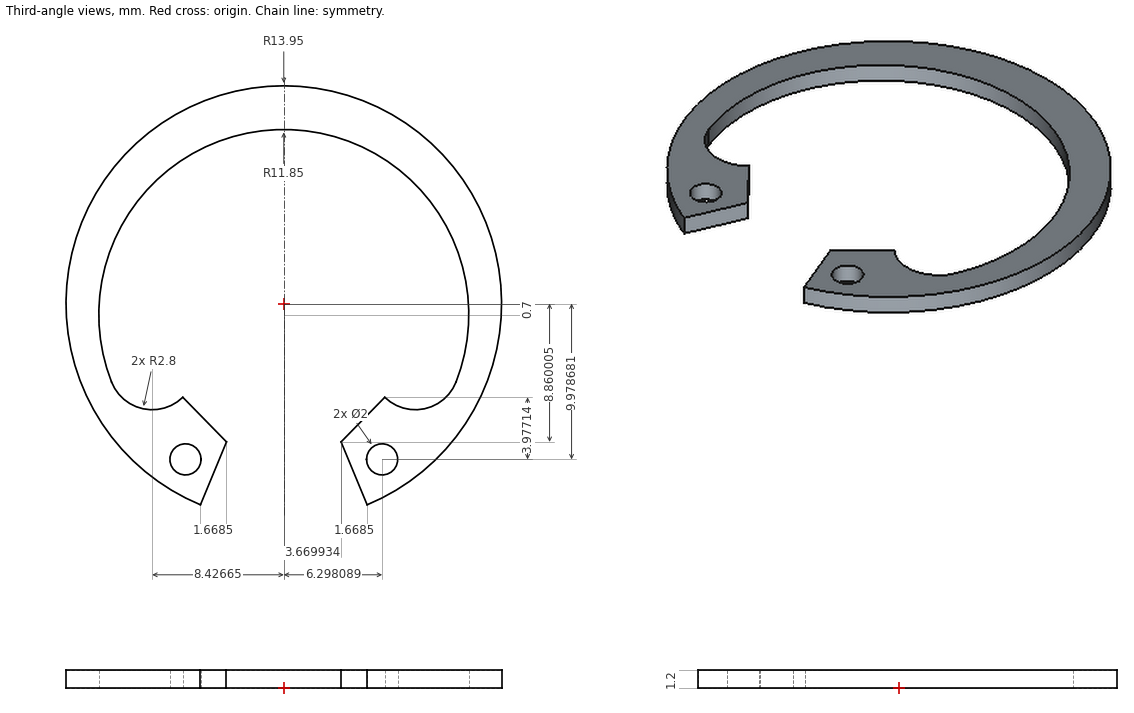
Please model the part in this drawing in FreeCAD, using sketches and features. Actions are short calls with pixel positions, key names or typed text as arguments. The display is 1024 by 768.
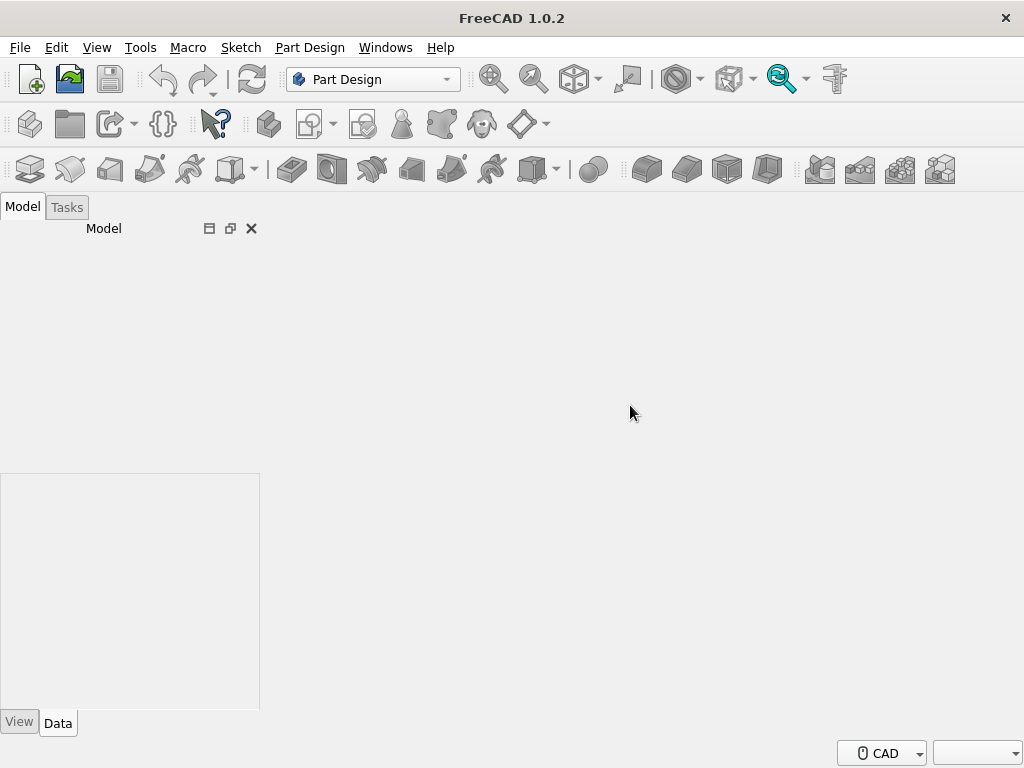
click(30, 80)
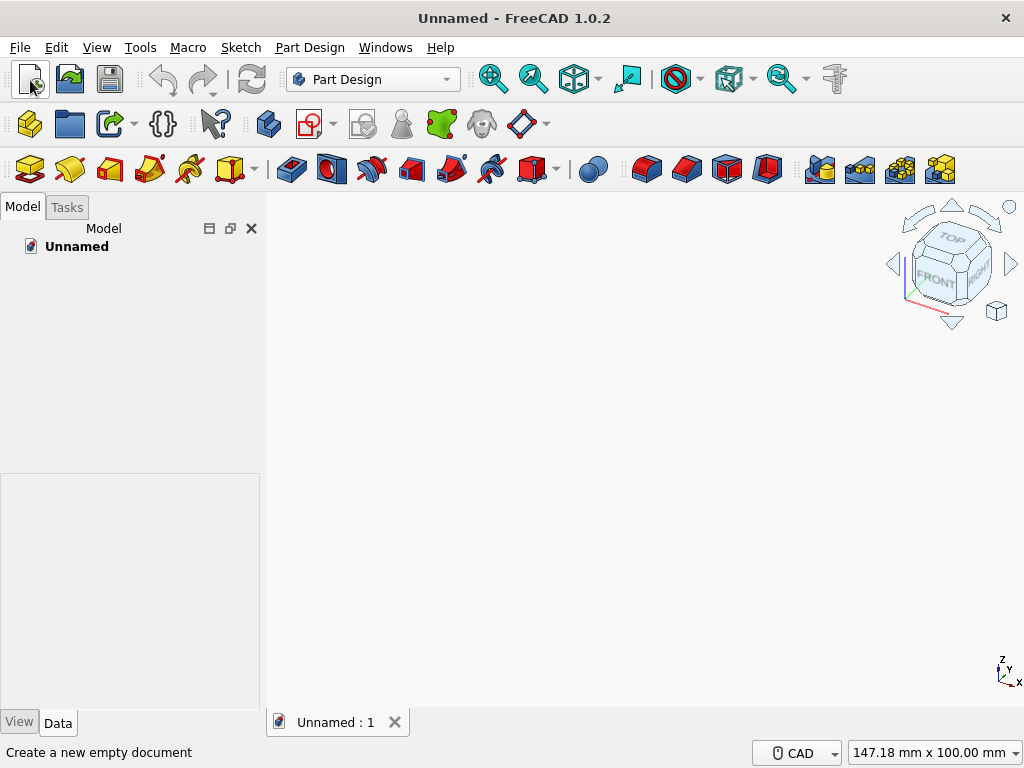
click(310, 124)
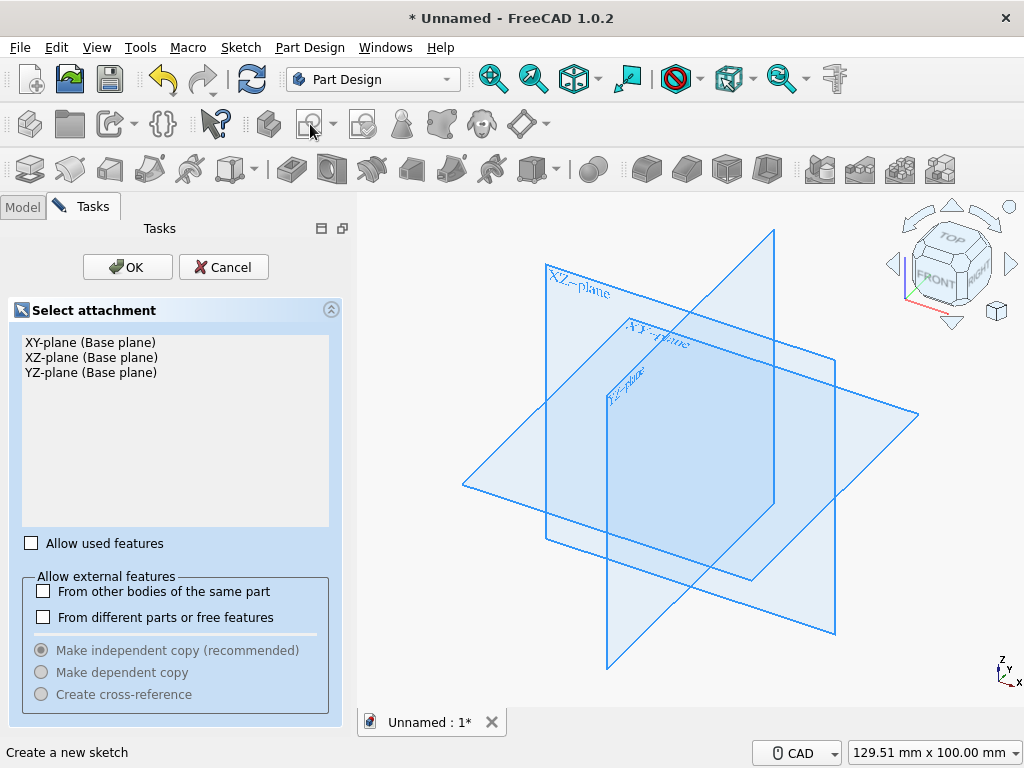
click(82, 342)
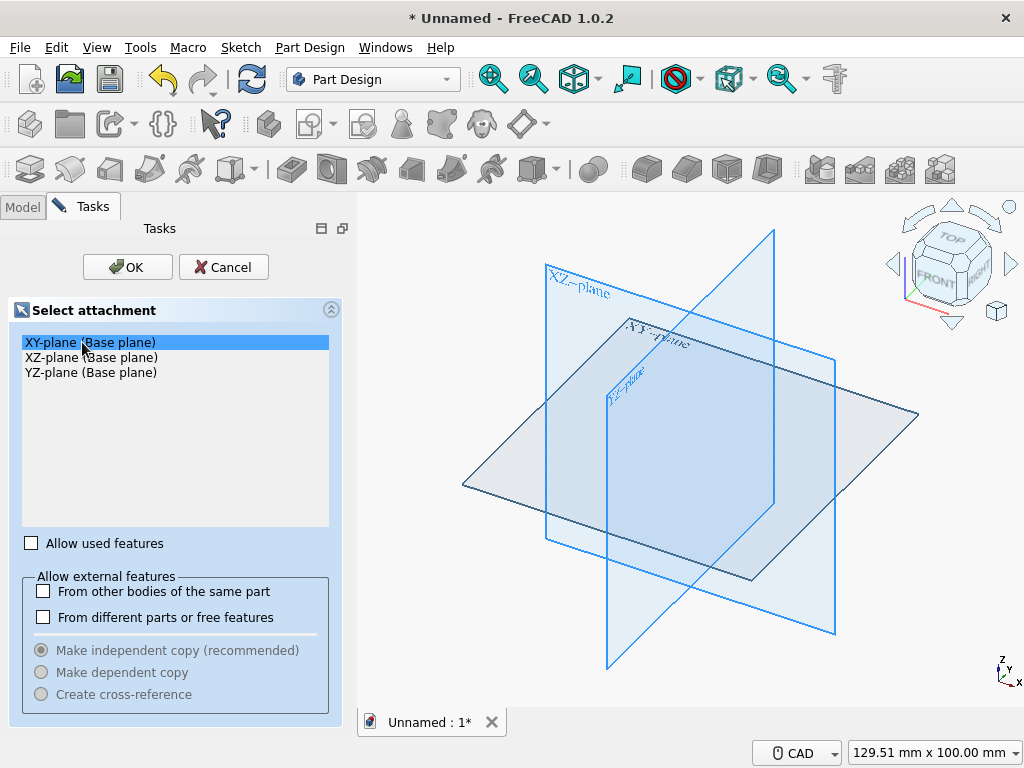
click(128, 267)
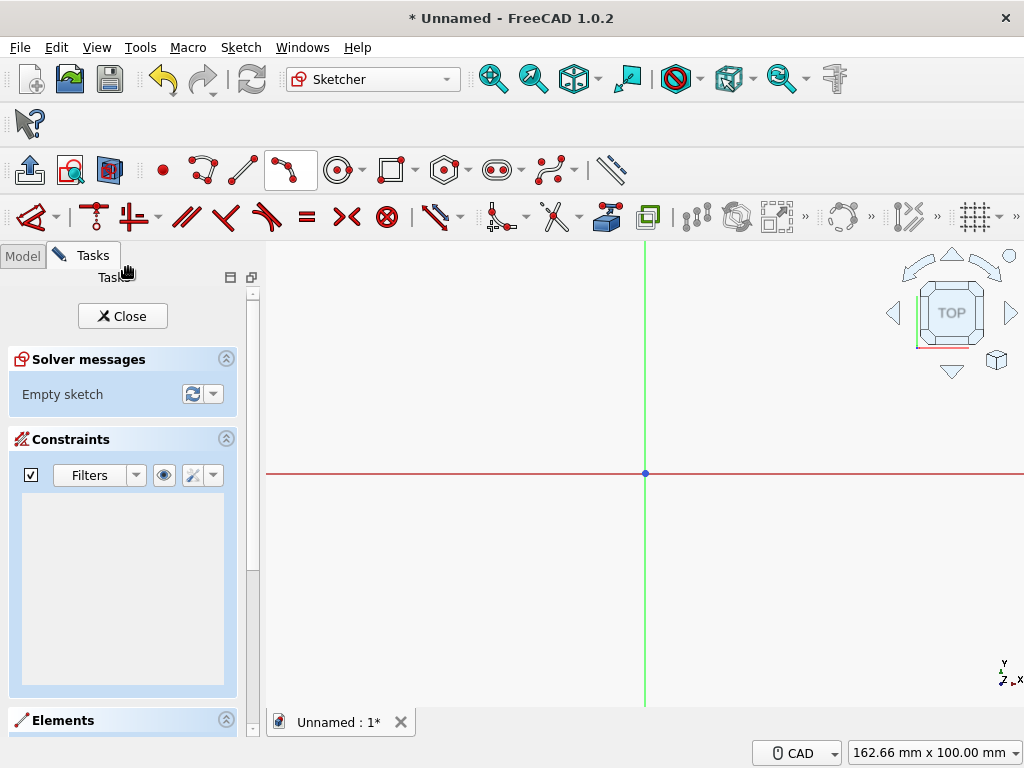
scroll(701, 470, up, 4)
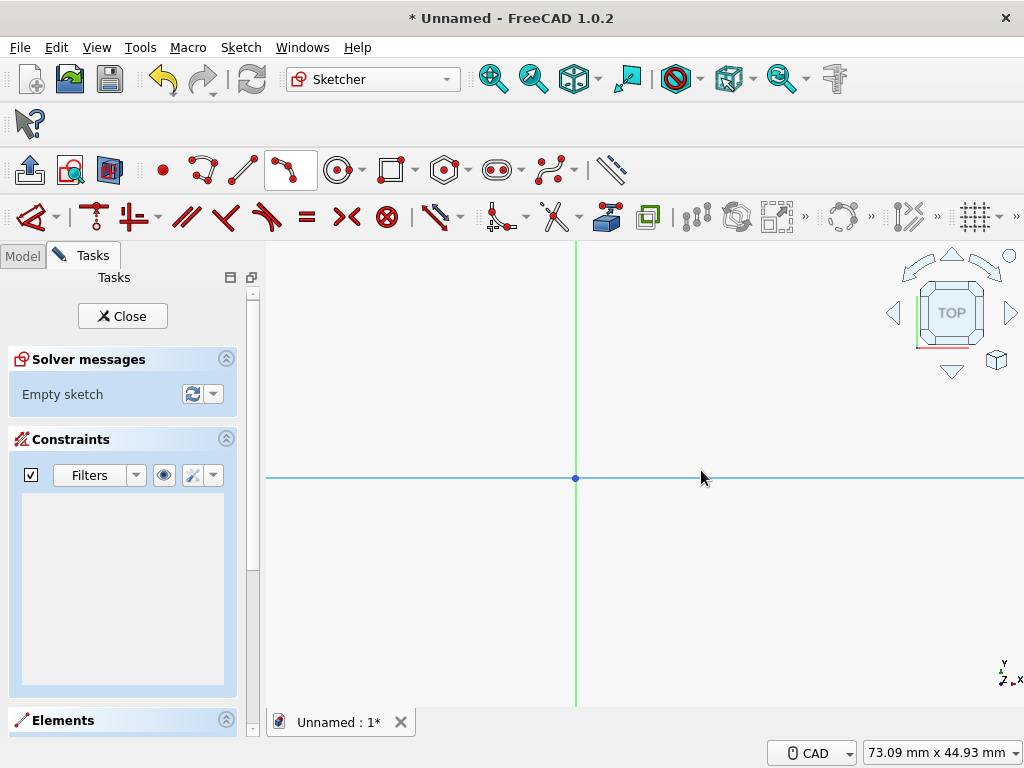
click(204, 170)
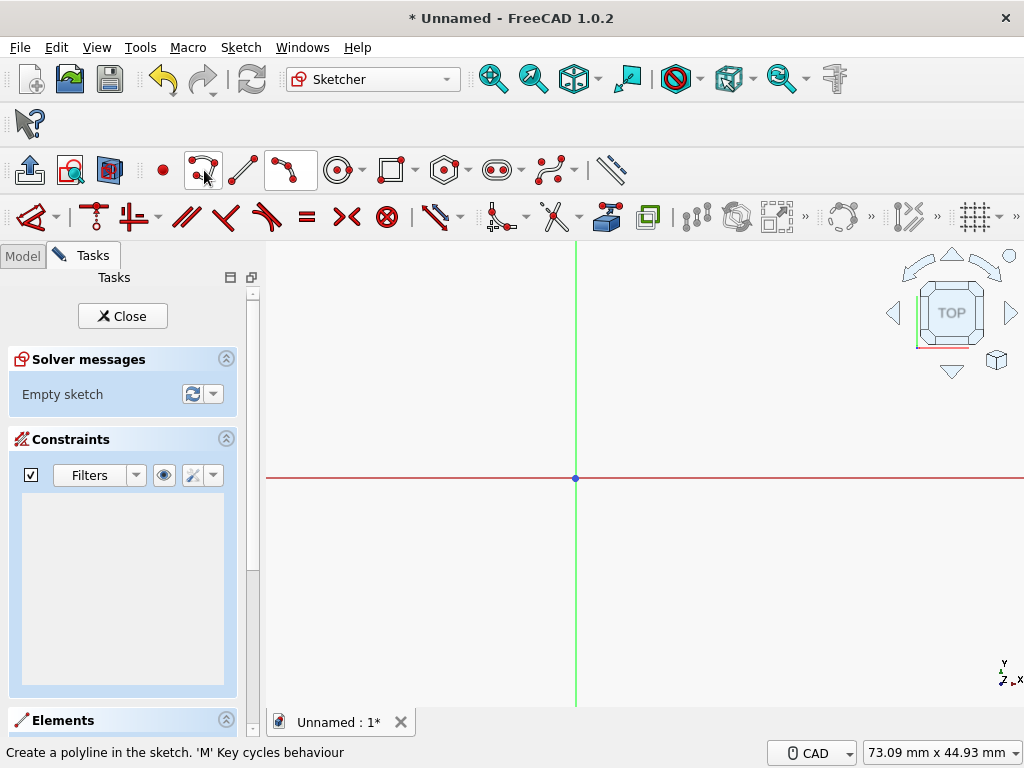
click(643, 541)
click(614, 570)
click(631, 612)
right_click(631, 612)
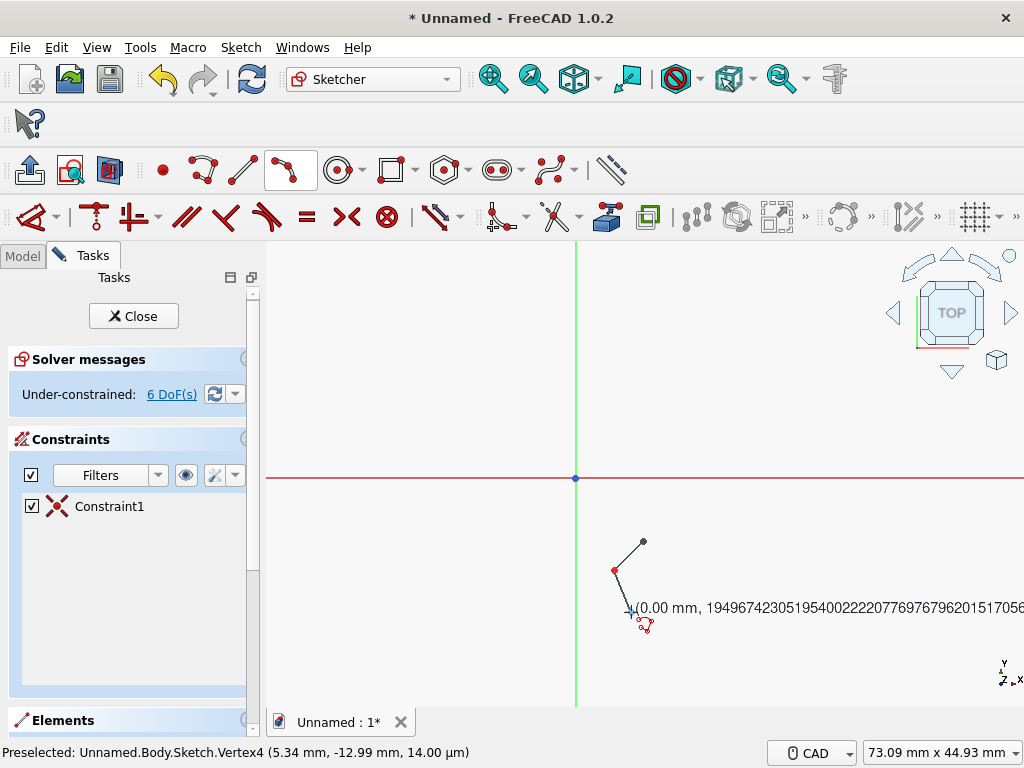
click(520, 612)
click(538, 570)
click(509, 541)
right_click(509, 541)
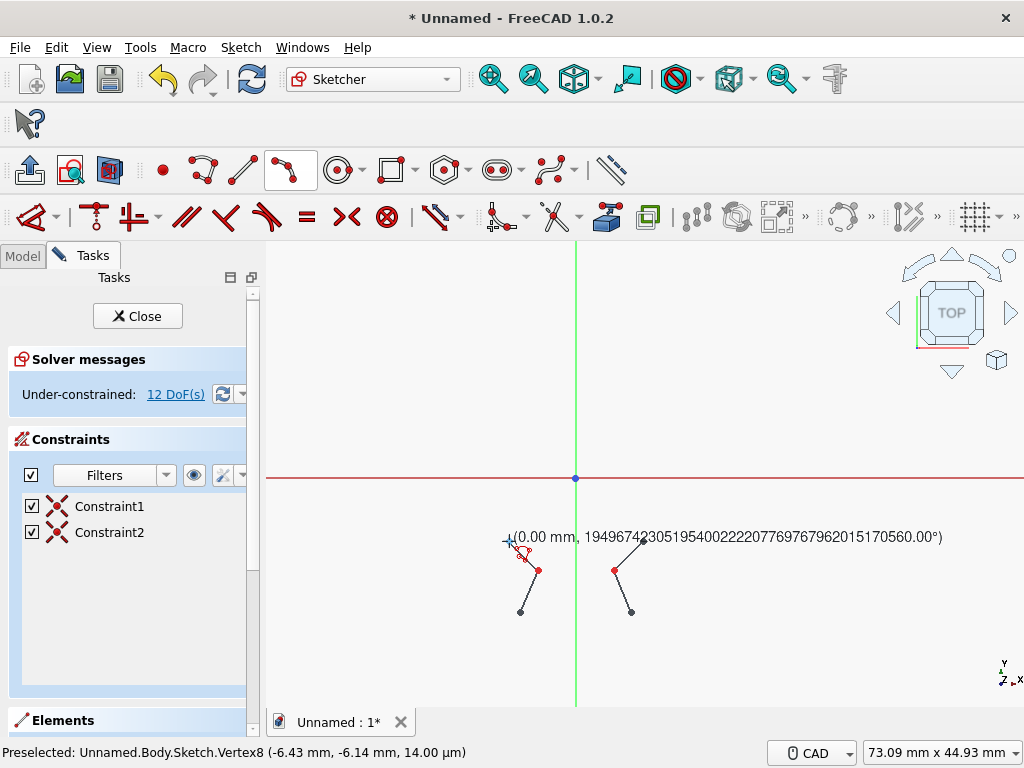
key(g)
key(3)
key(a)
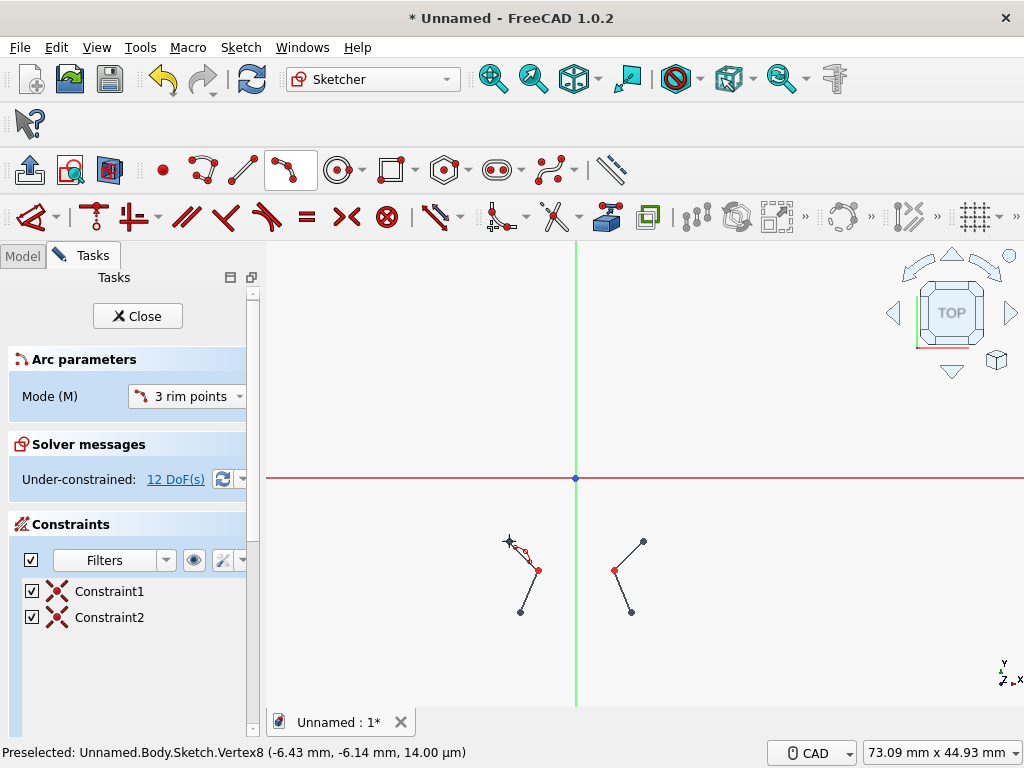
click(631, 613)
click(520, 613)
click(651, 355)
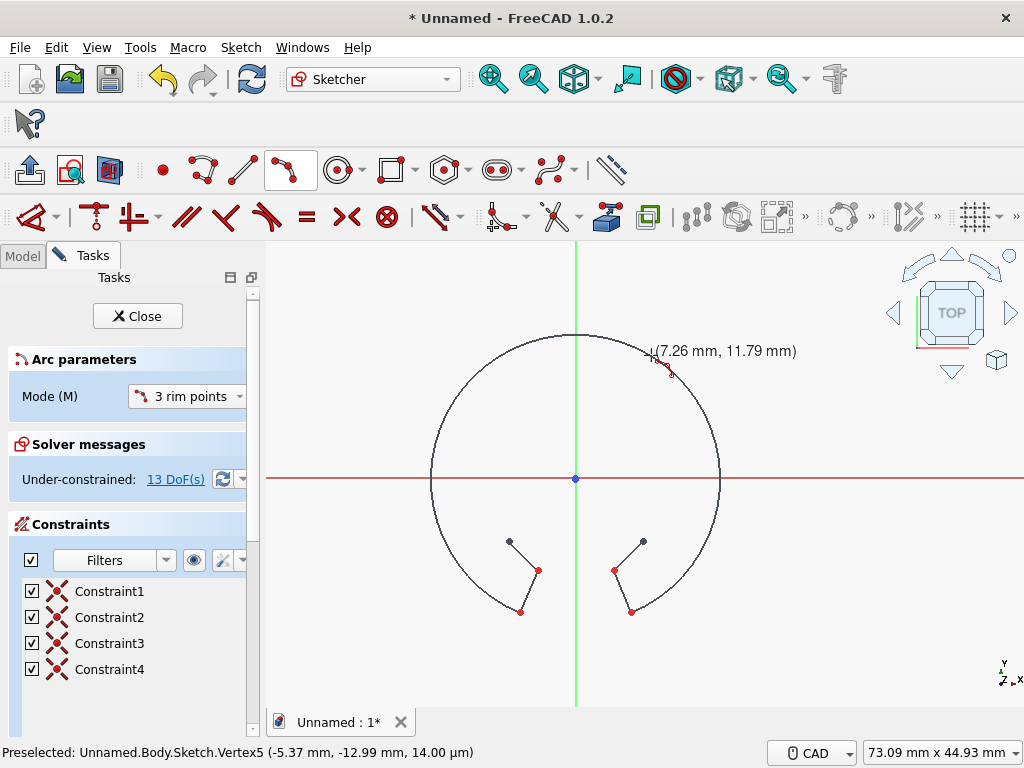
click(509, 542)
click(461, 530)
click(482, 548)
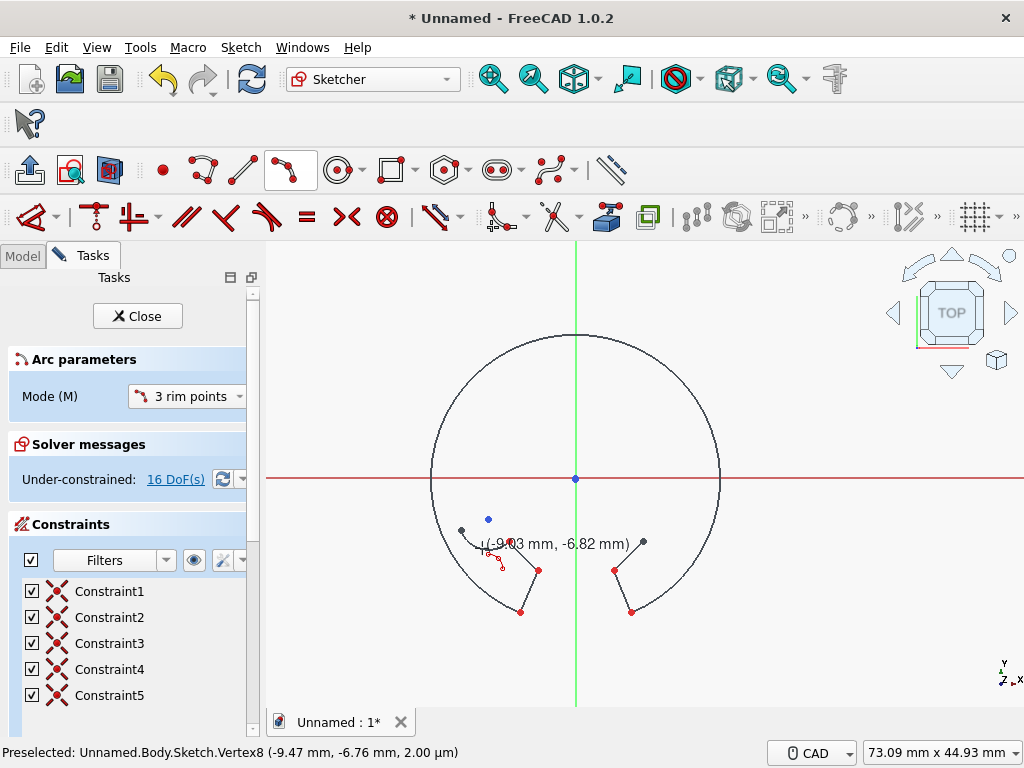
click(461, 531)
click(690, 530)
click(622, 372)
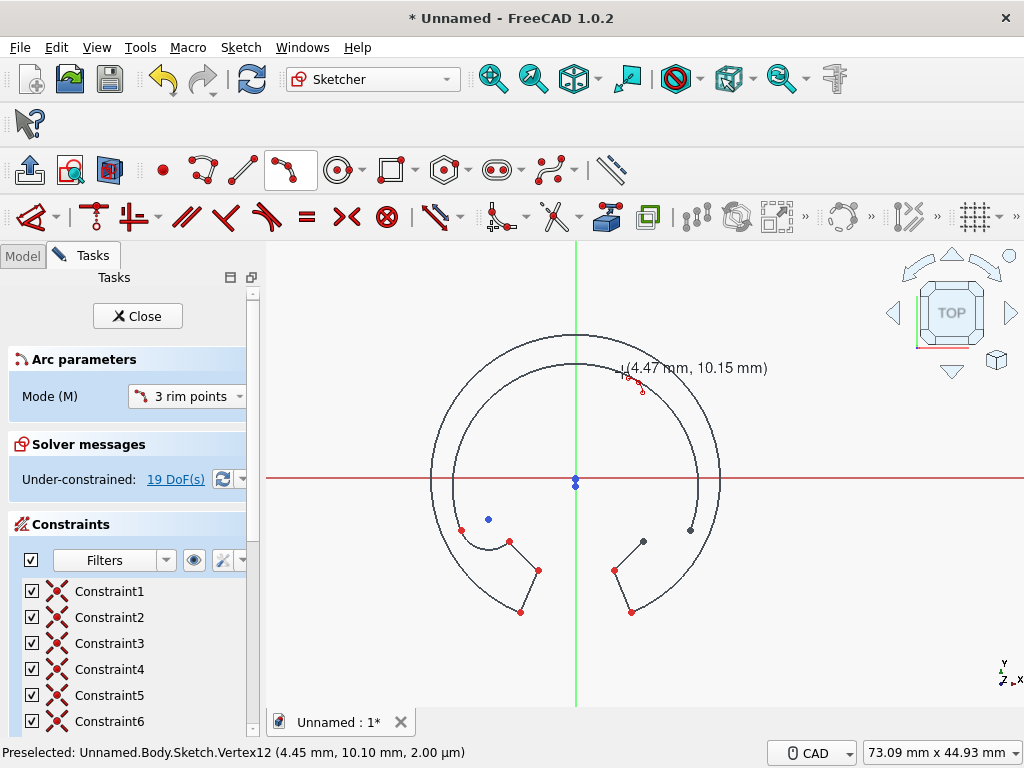
click(690, 531)
click(643, 542)
click(669, 548)